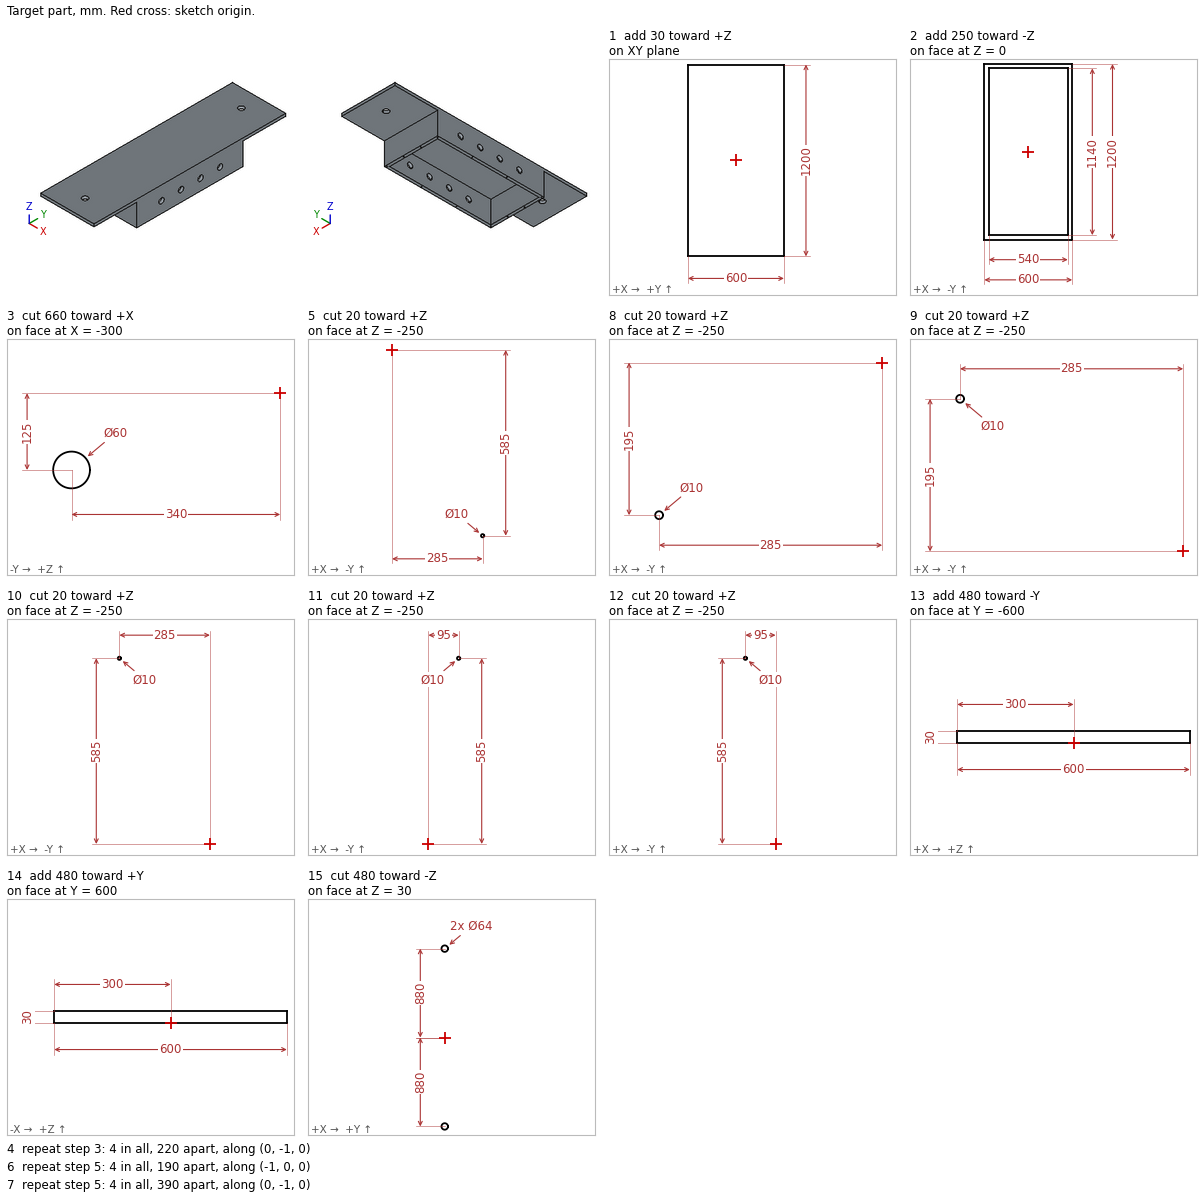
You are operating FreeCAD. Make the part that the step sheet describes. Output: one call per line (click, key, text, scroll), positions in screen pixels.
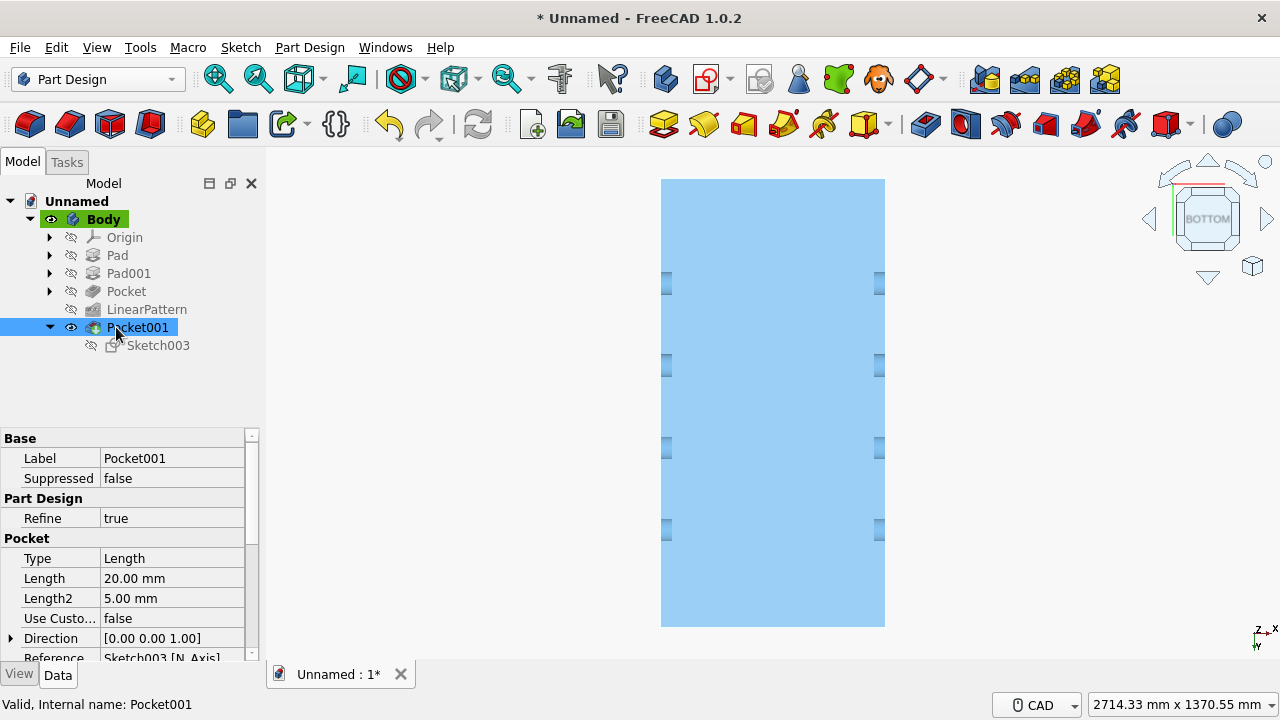
click(1026, 80)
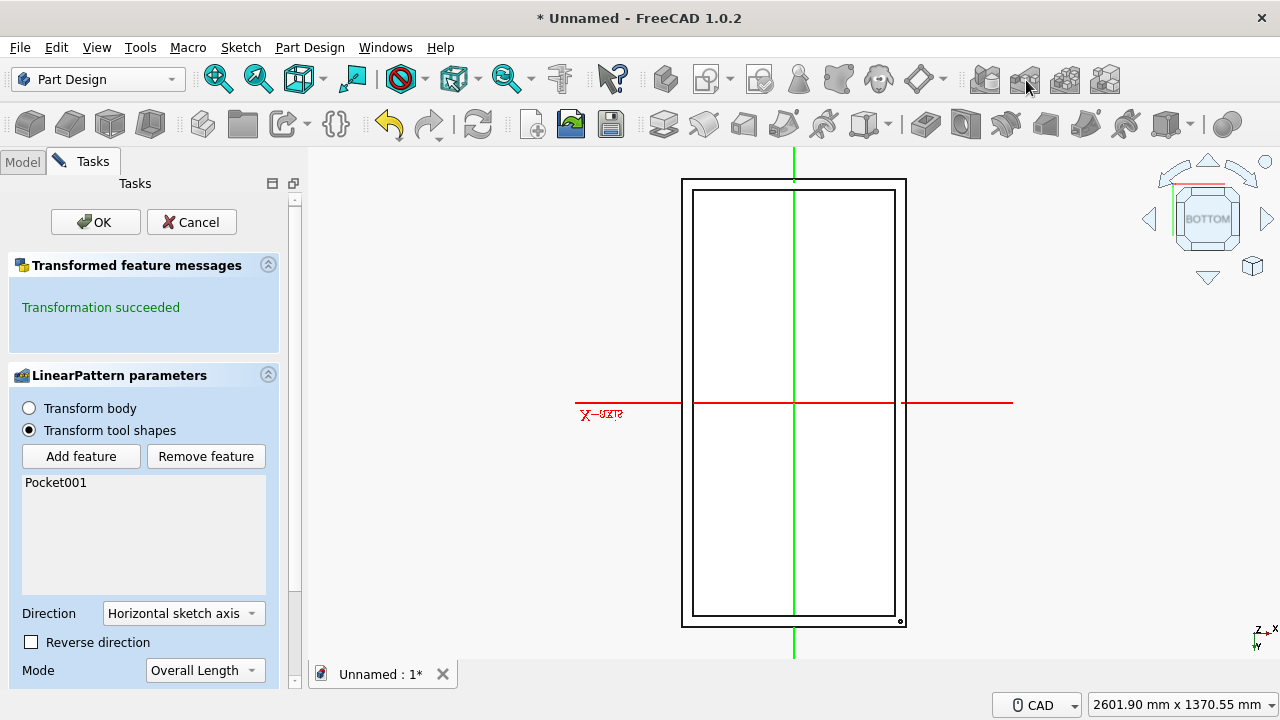
click(184, 614)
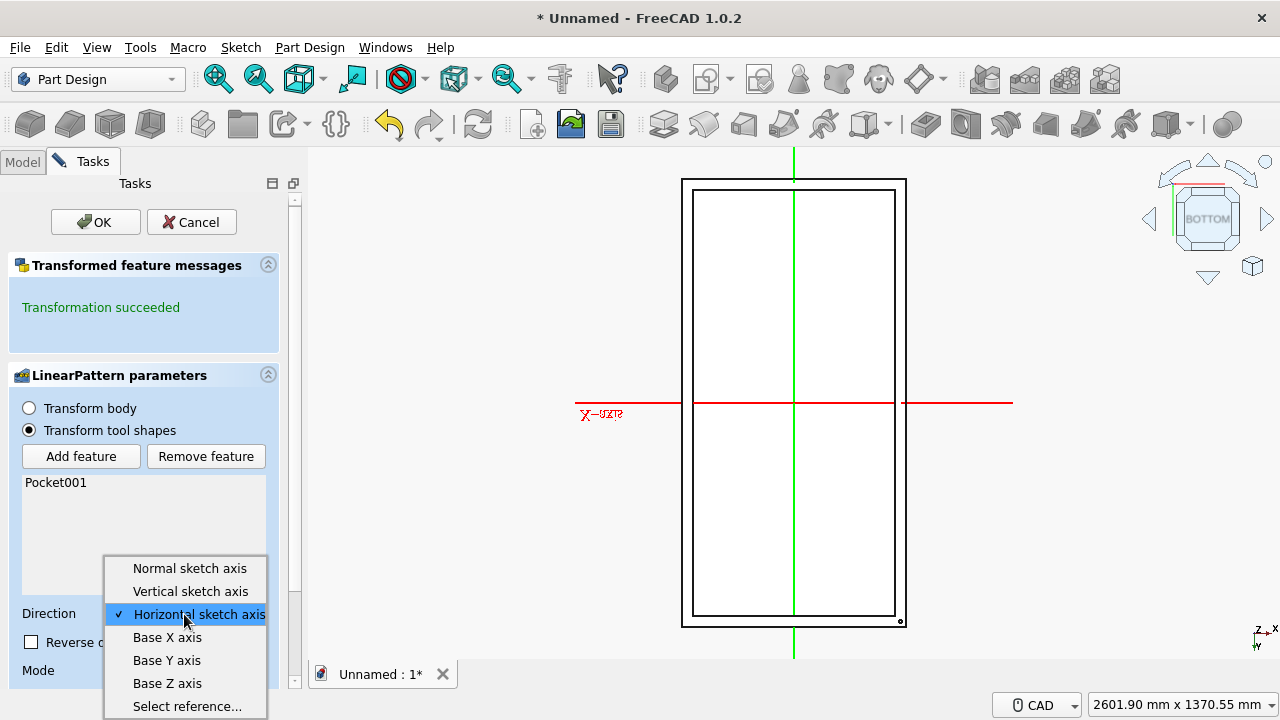
click(184, 638)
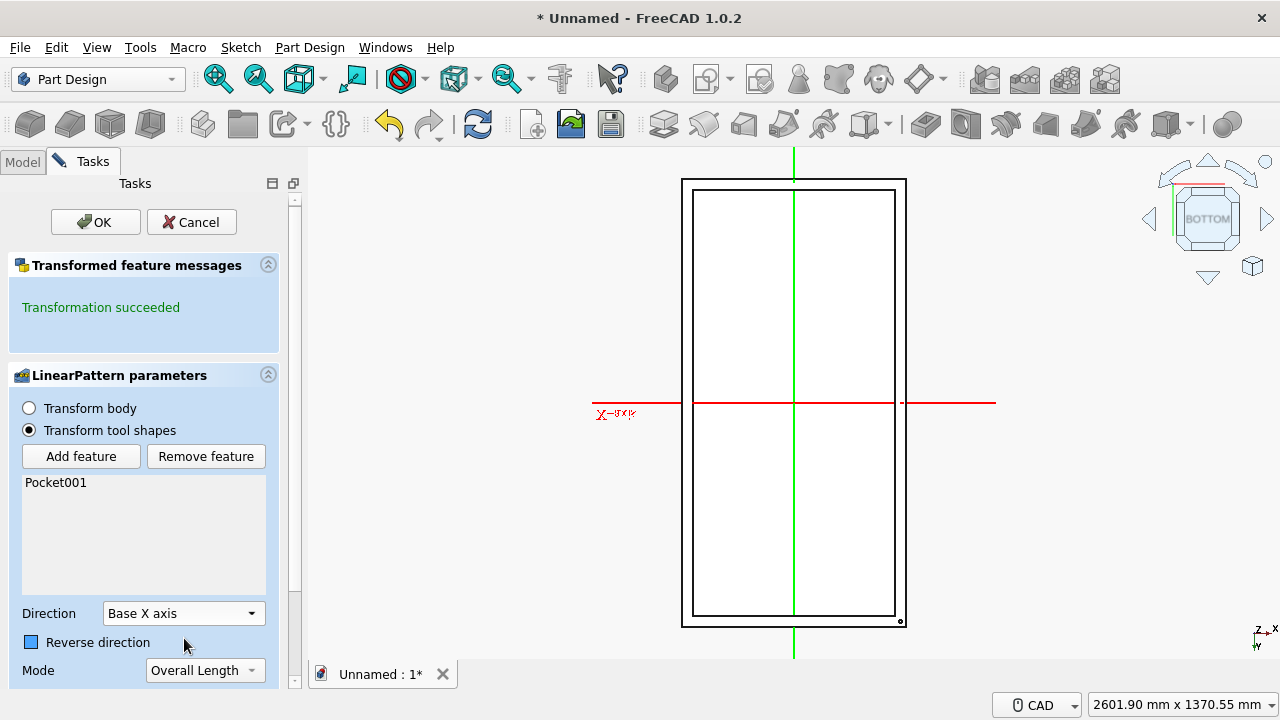
click(206, 670)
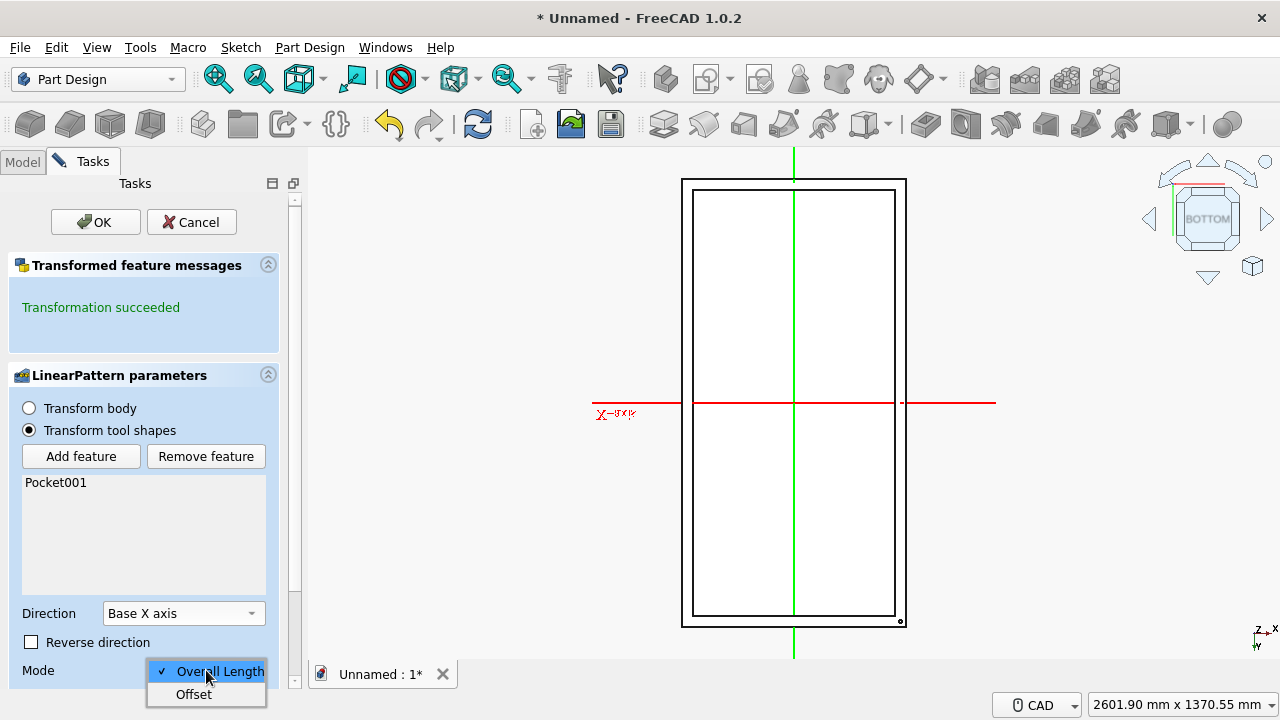
click(206, 694)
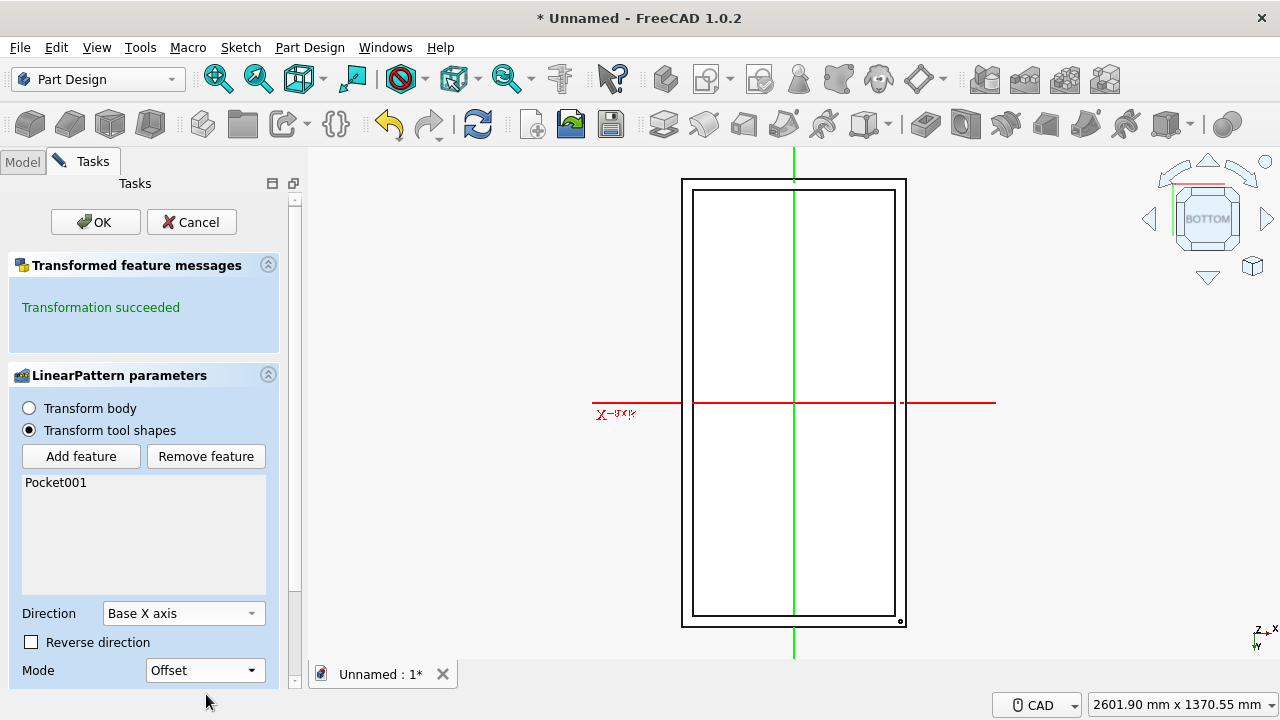
scroll(295, 440, down, 2)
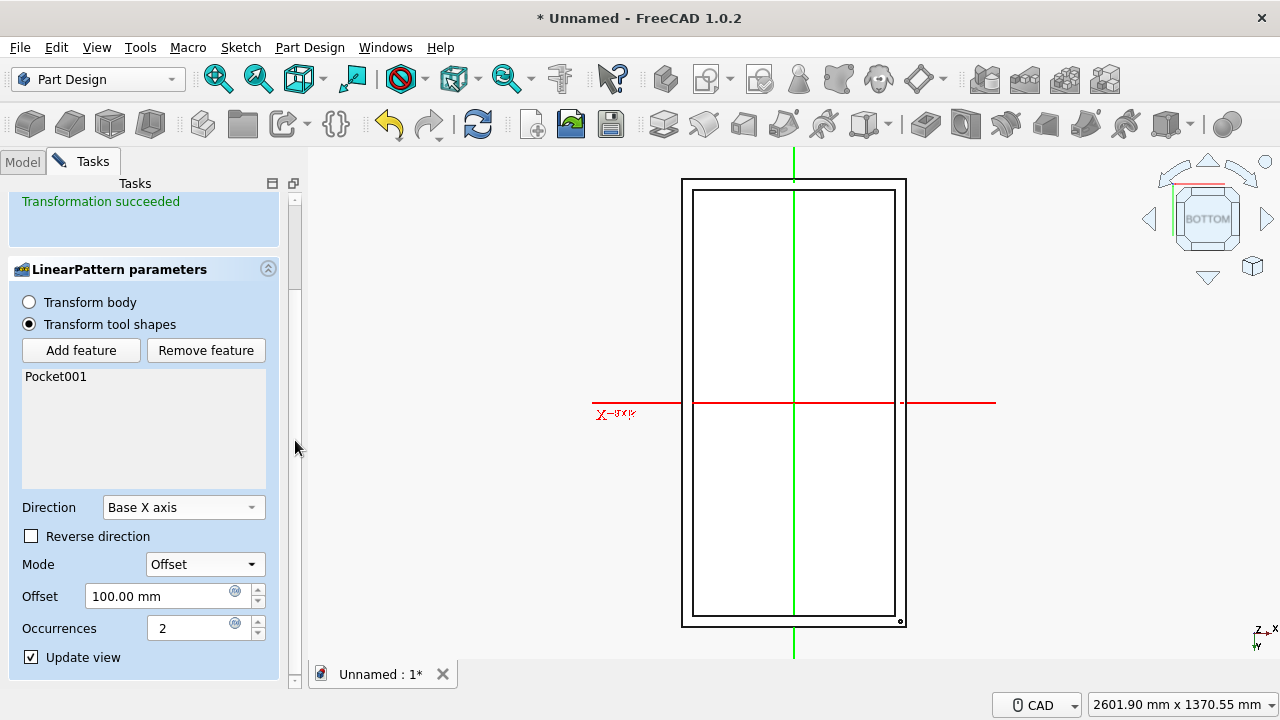
triple_click(168, 596)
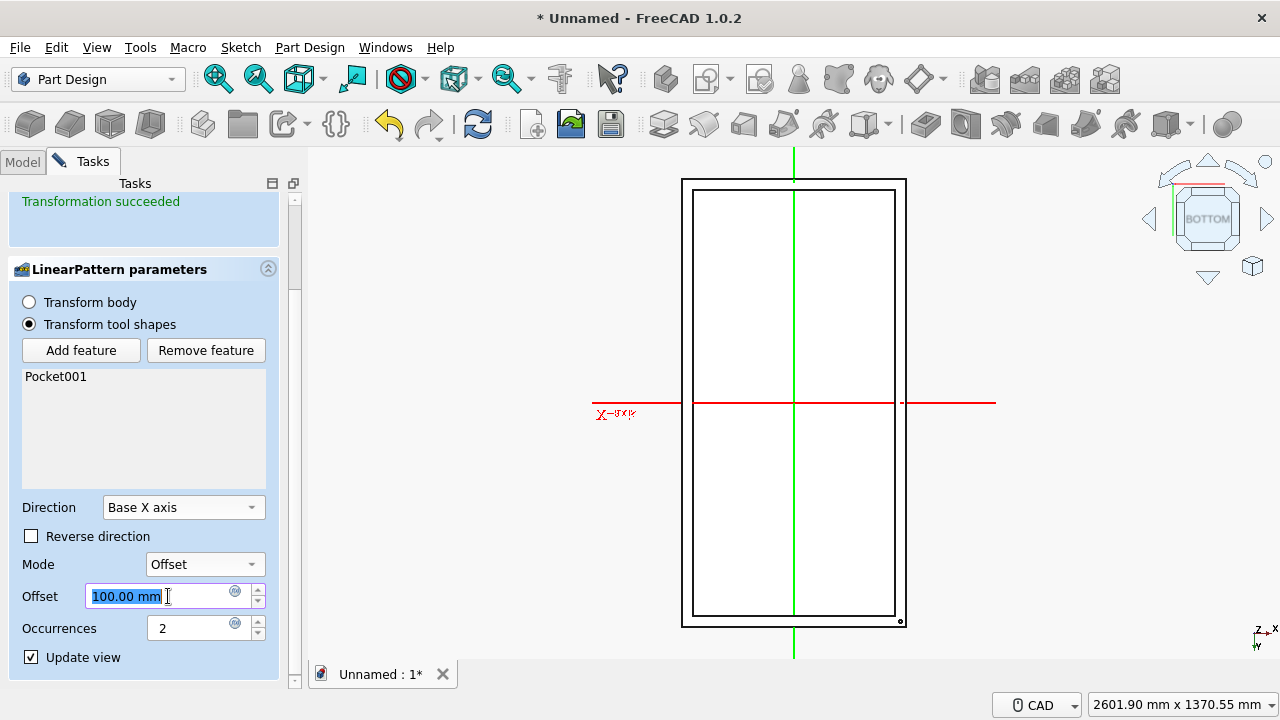
text(190)
key(Tab)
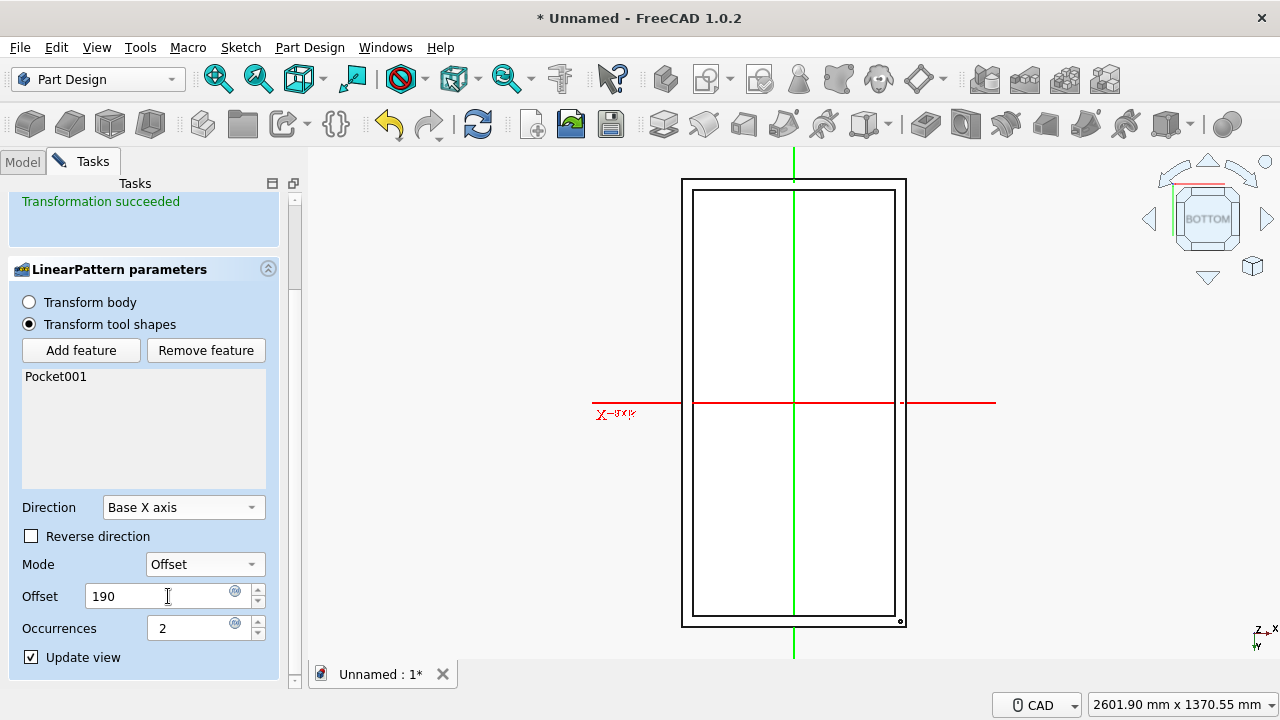
triple_click(198, 628)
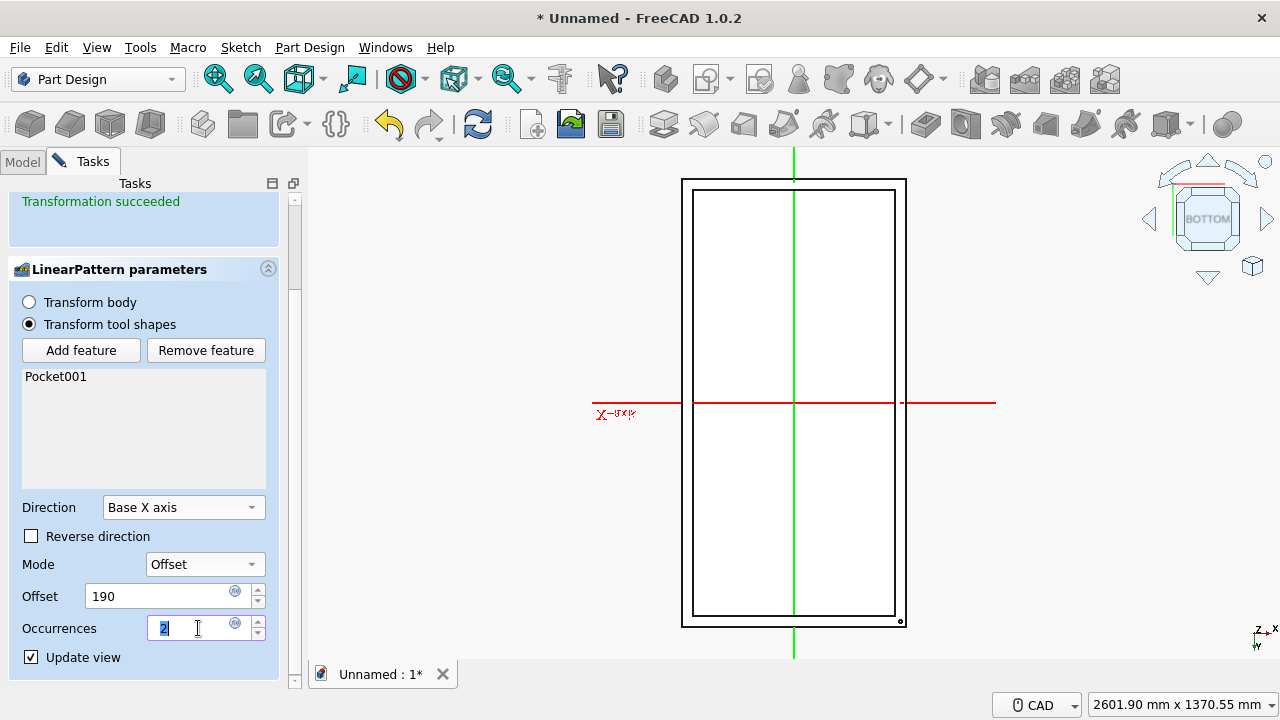
text(4)
key(Tab)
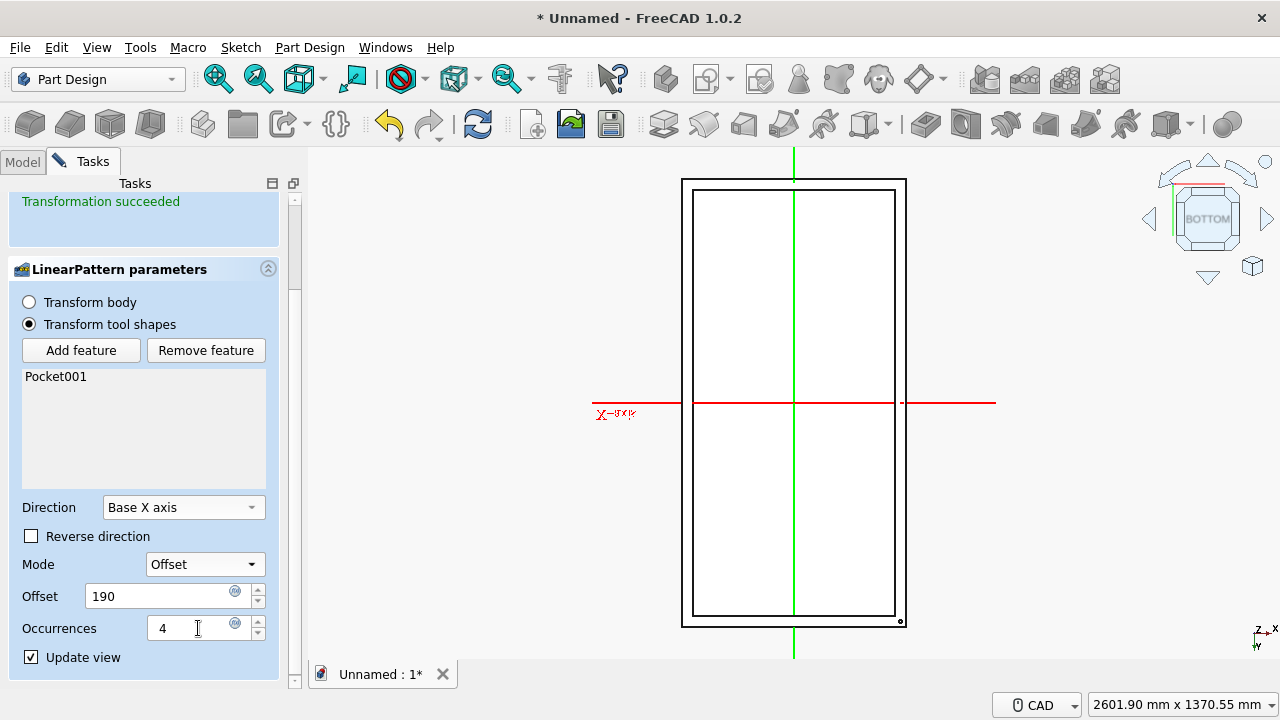
click(30, 536)